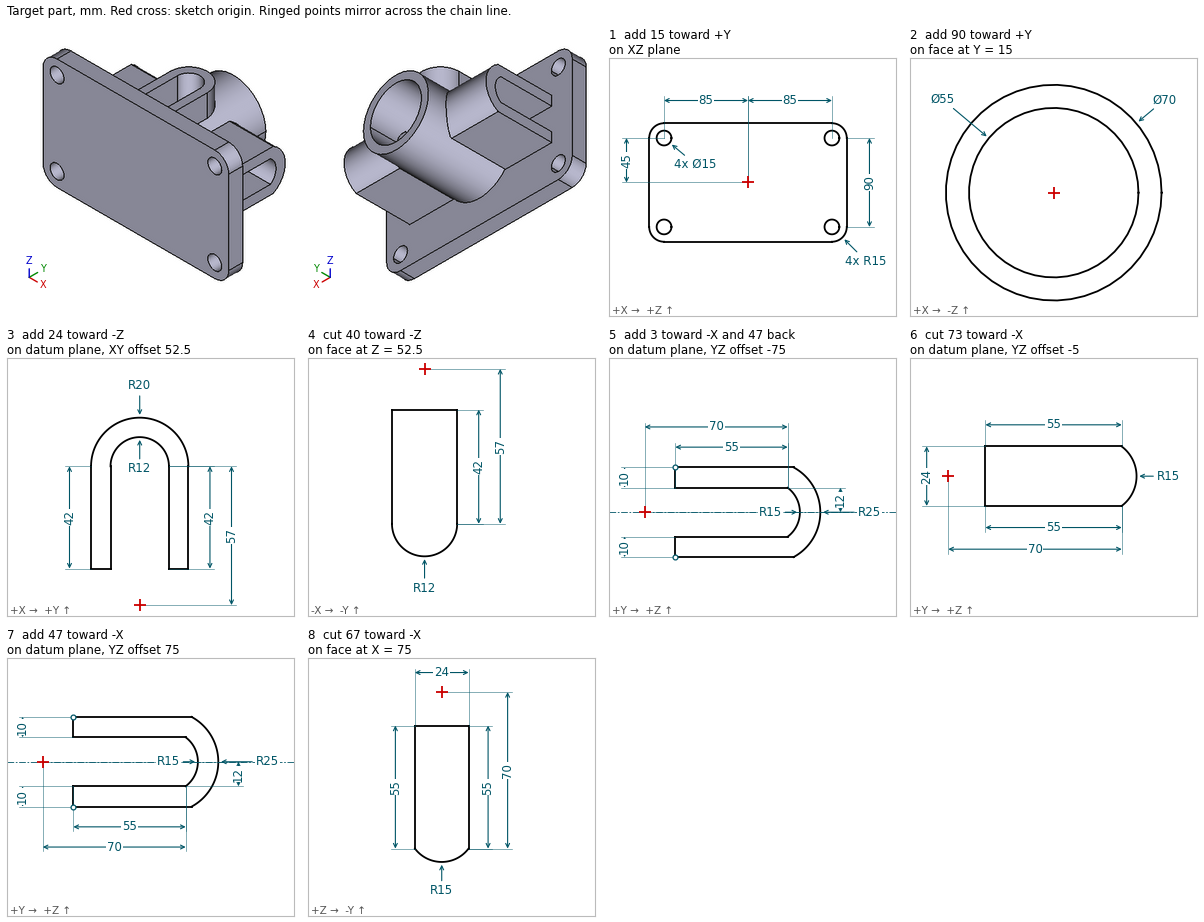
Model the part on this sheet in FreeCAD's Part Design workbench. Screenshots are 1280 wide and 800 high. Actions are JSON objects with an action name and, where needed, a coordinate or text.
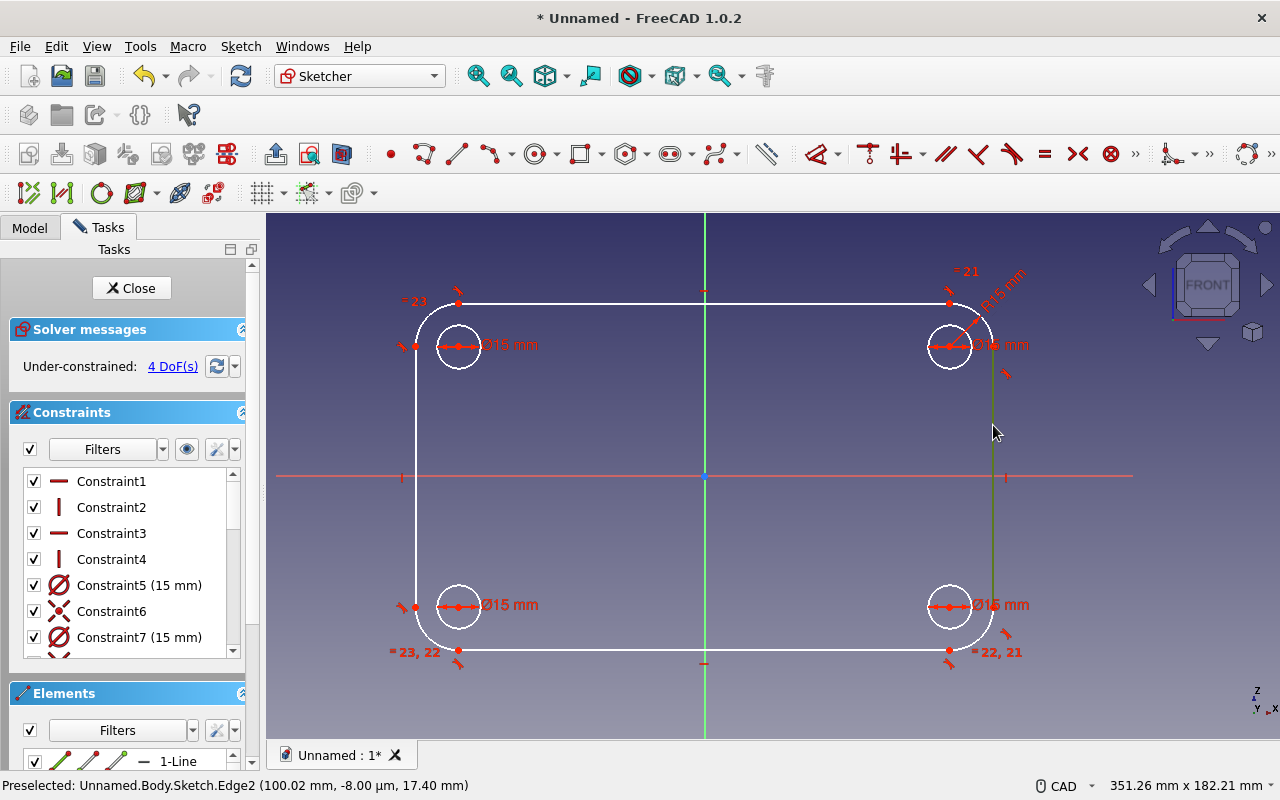
{"action": "key", "text": "i"}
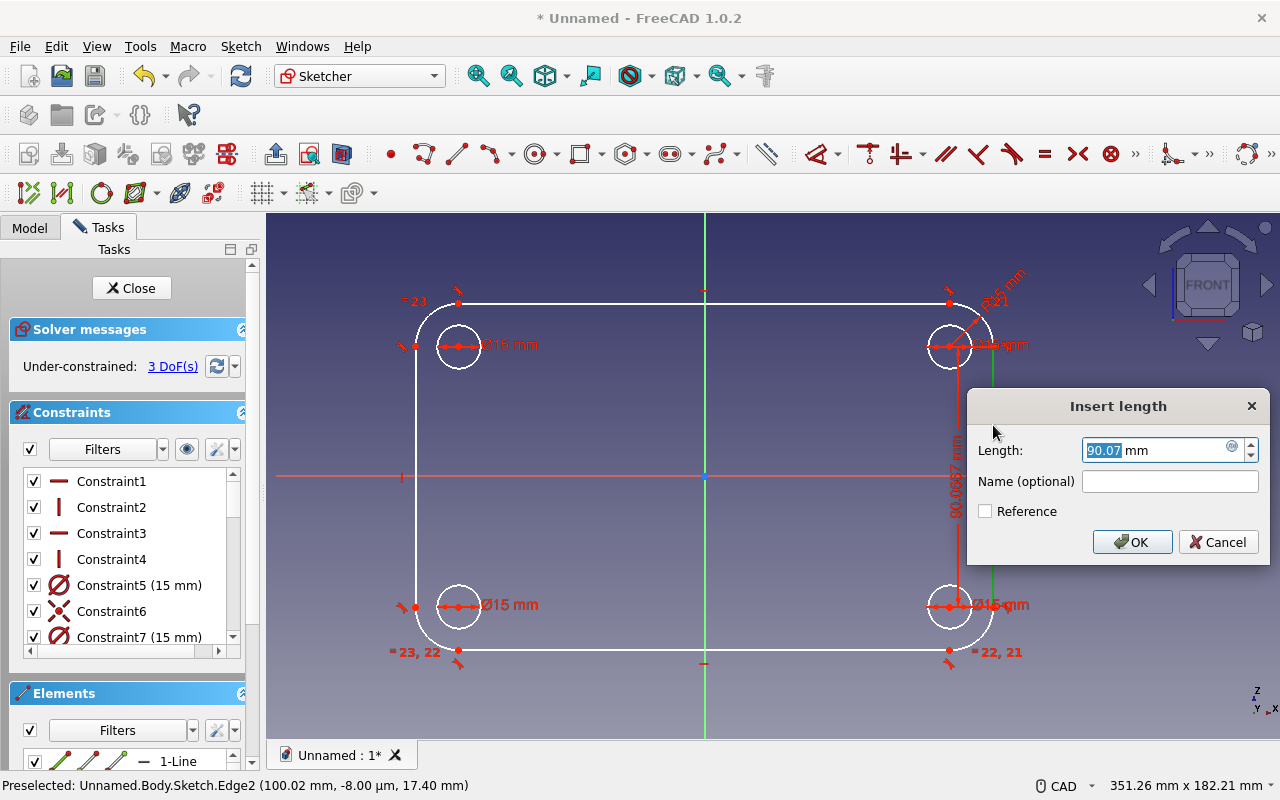
{"action": "type", "text": "90"}
{"action": "key", "text": "Return"}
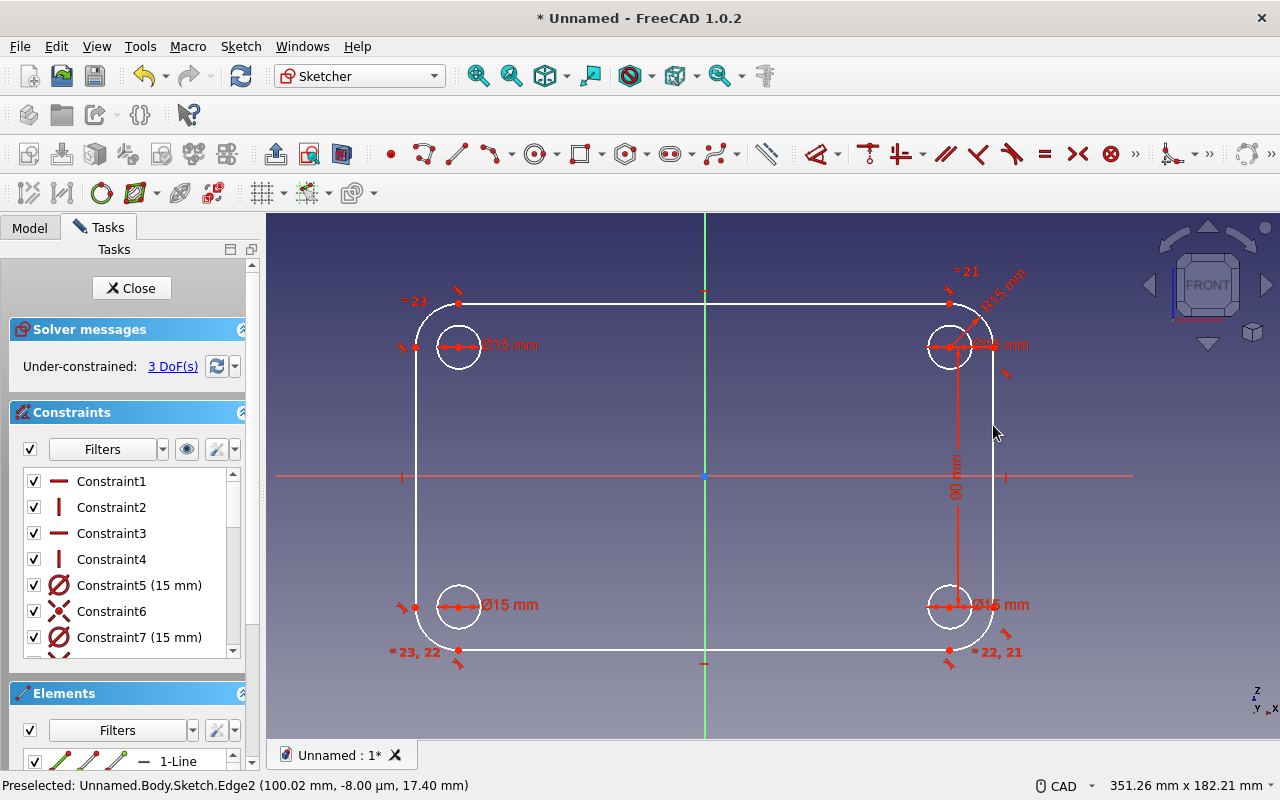
{"action": "left_click", "coordinate": [459, 347]}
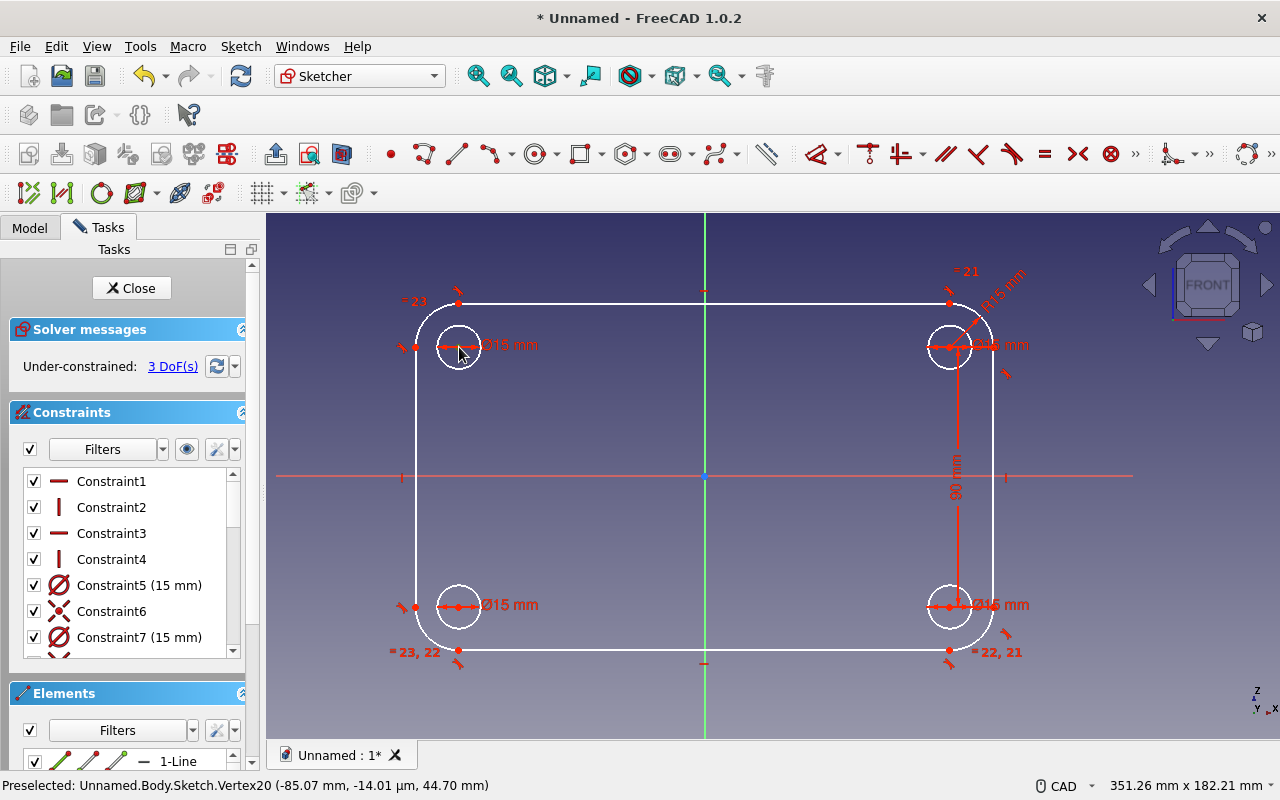
{"action": "key", "text": "l"}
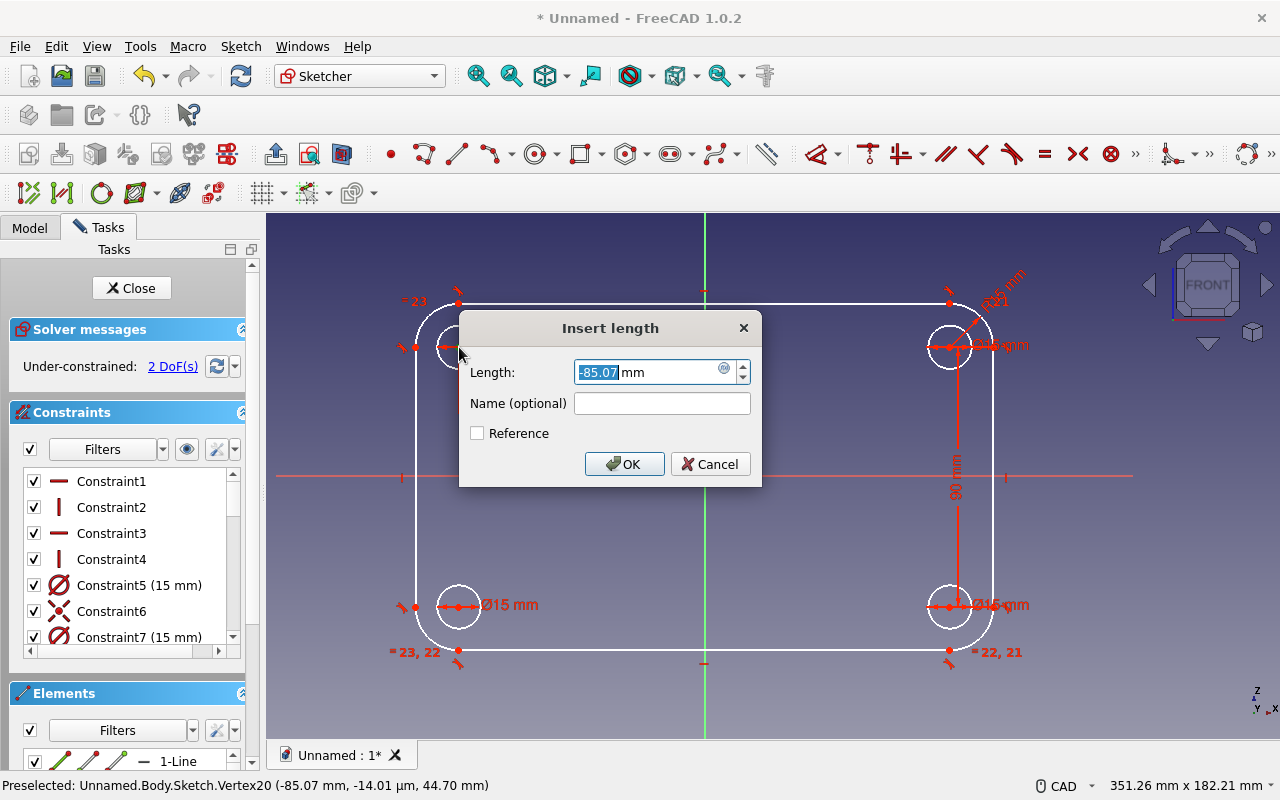
{"action": "type", "text": "-85"}
{"action": "key", "text": "Return"}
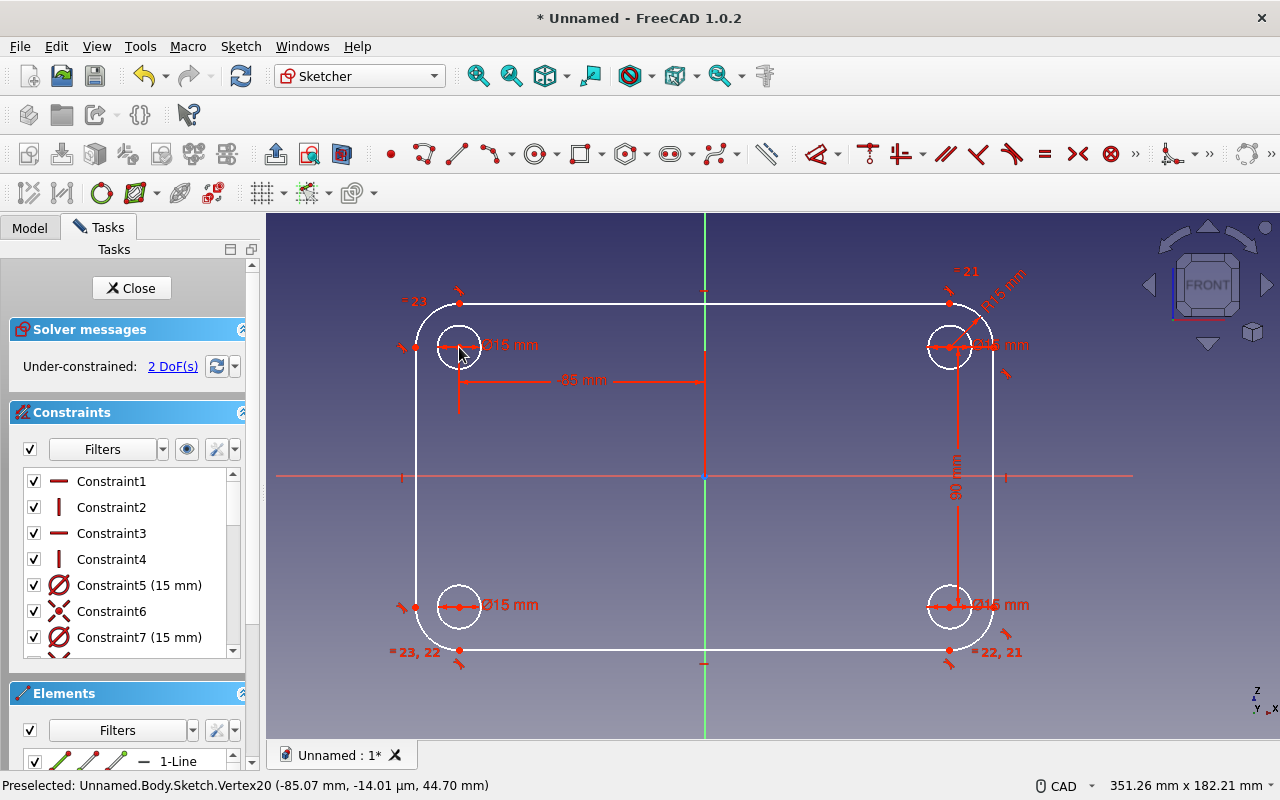
{"action": "left_click", "coordinate": [459, 347]}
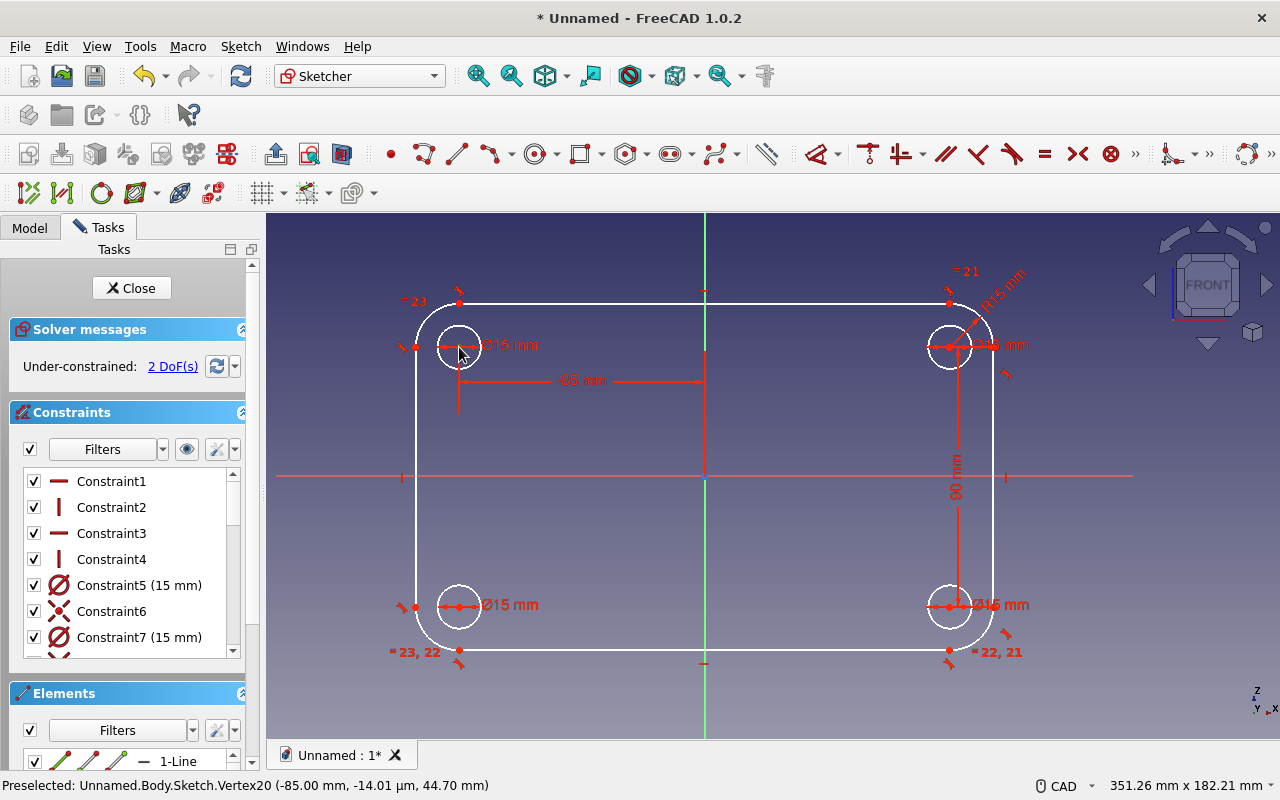
{"action": "key", "text": "i"}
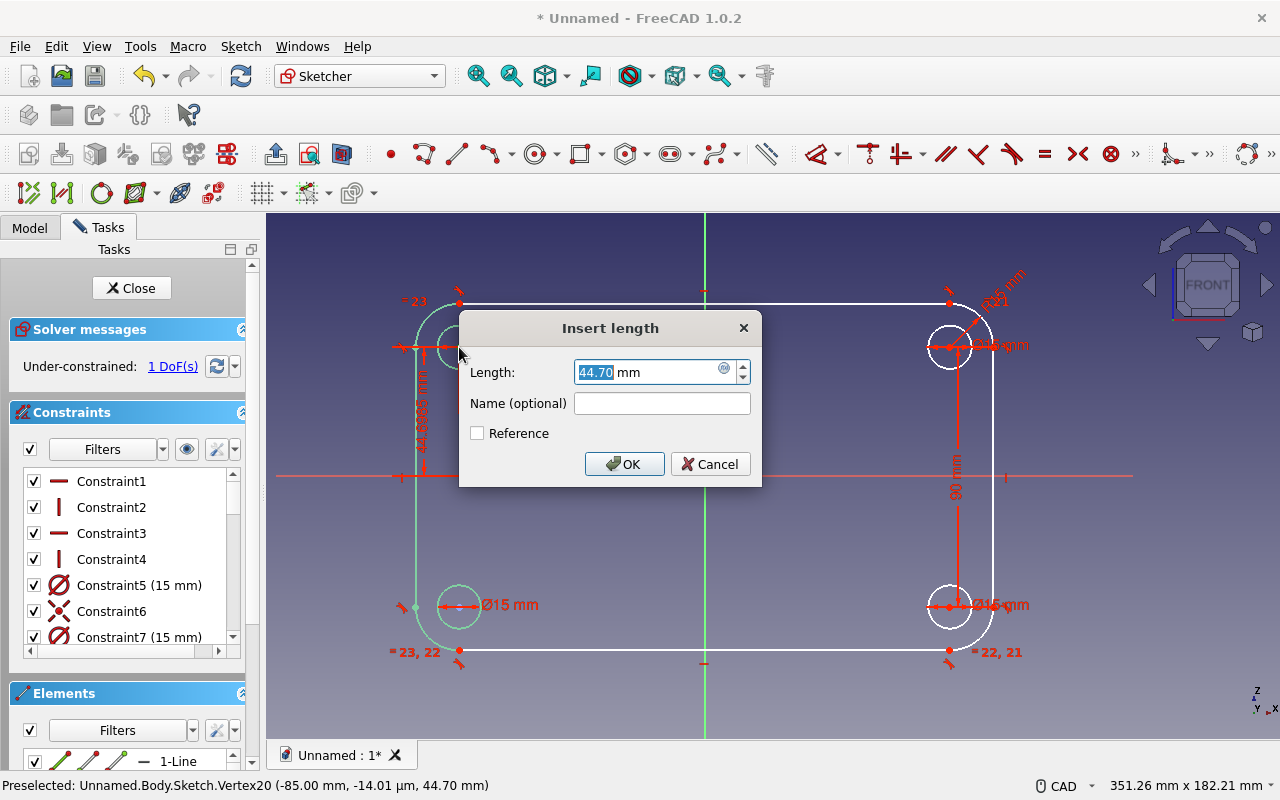
{"action": "type", "text": "45"}
{"action": "key", "text": "Return"}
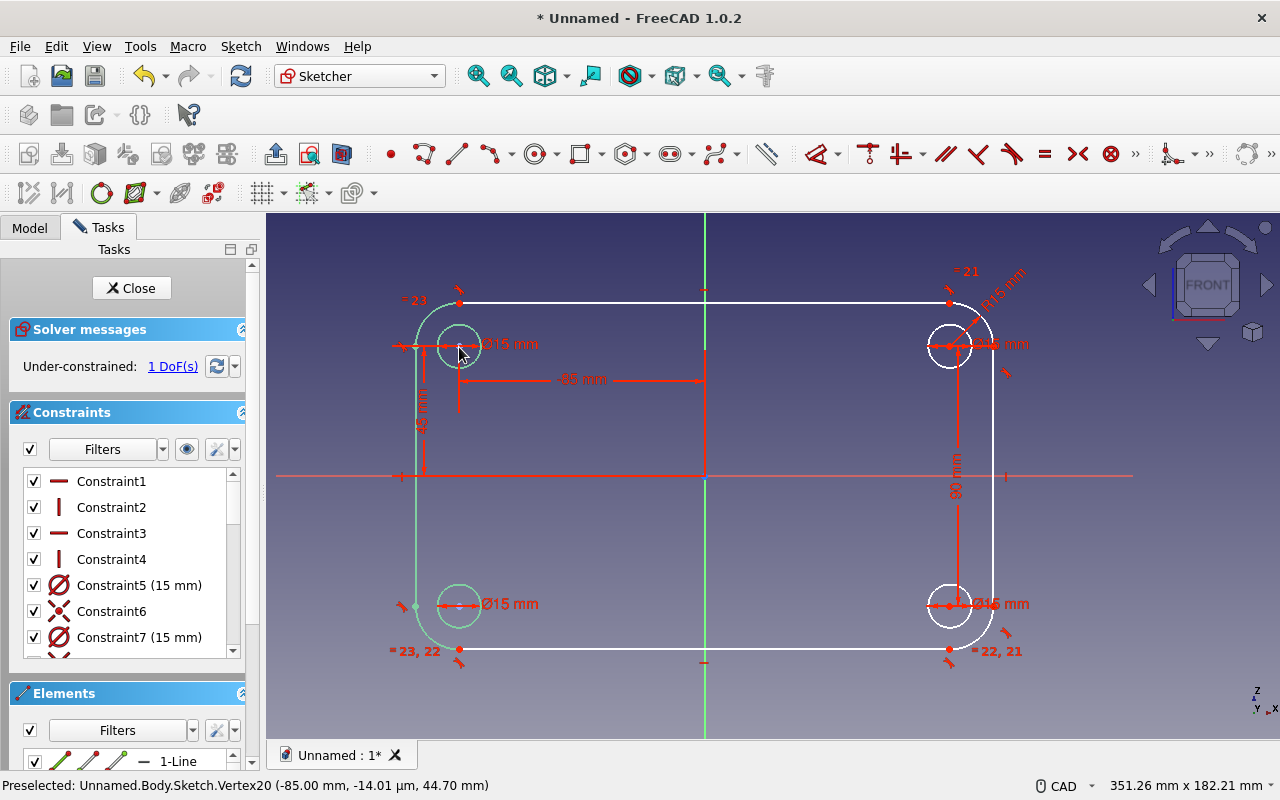
{"action": "left_click", "coordinate": [950, 346]}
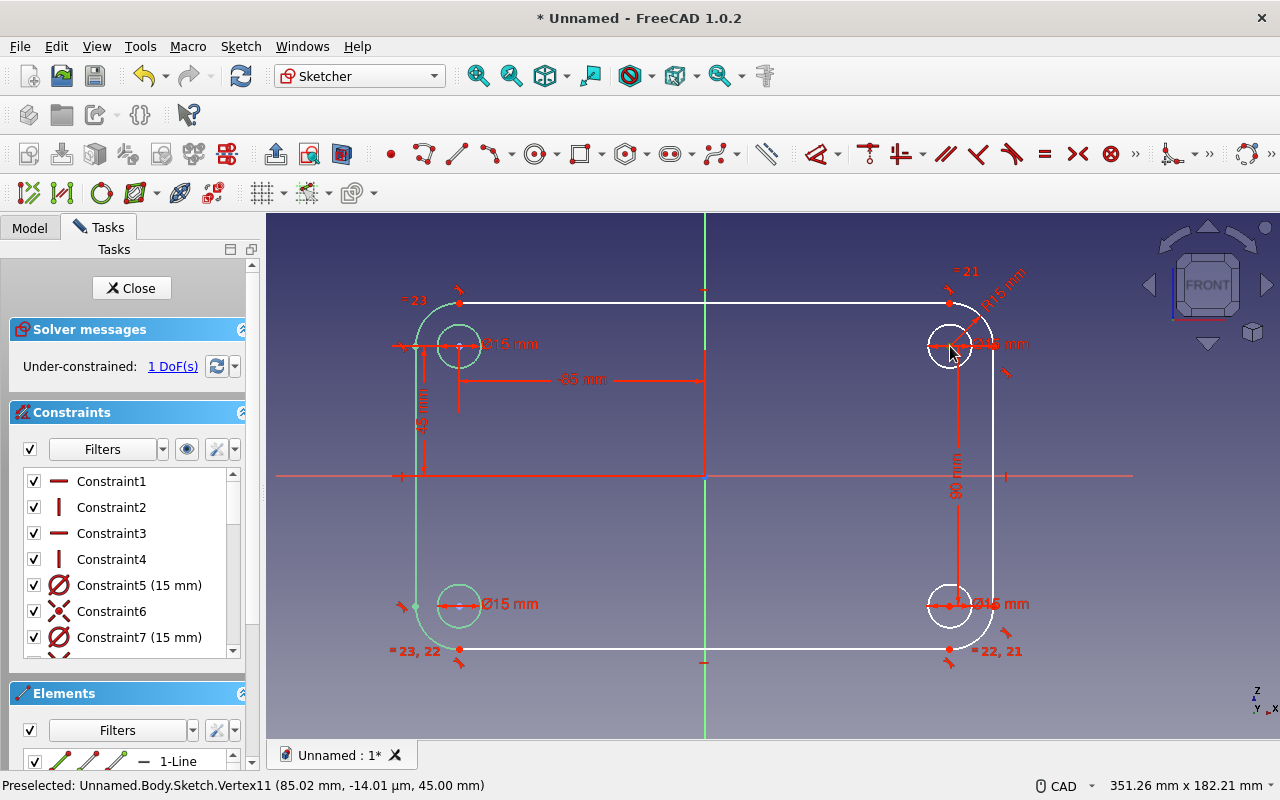
{"action": "key", "text": "l"}